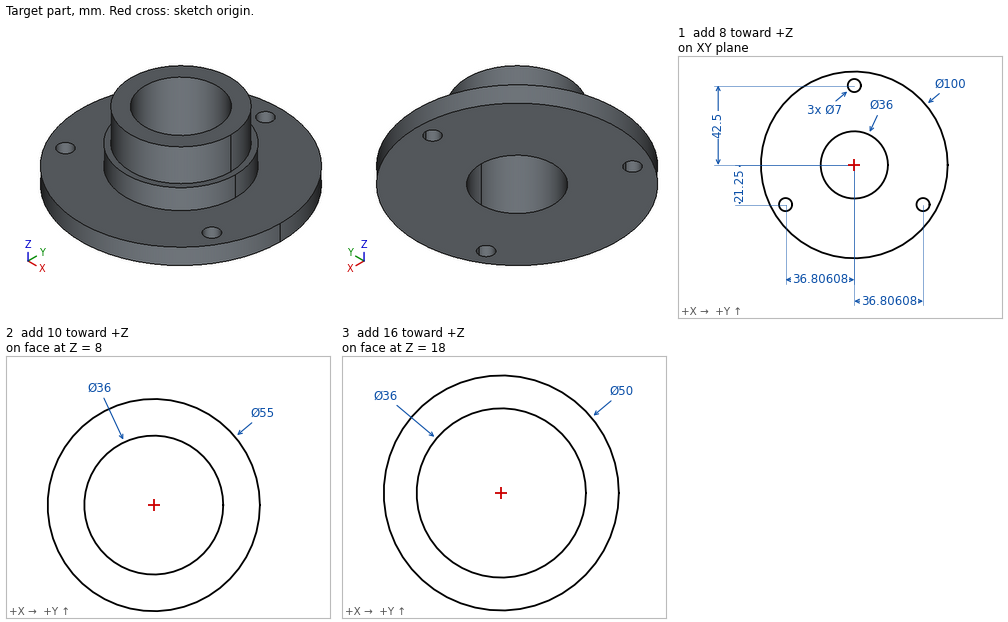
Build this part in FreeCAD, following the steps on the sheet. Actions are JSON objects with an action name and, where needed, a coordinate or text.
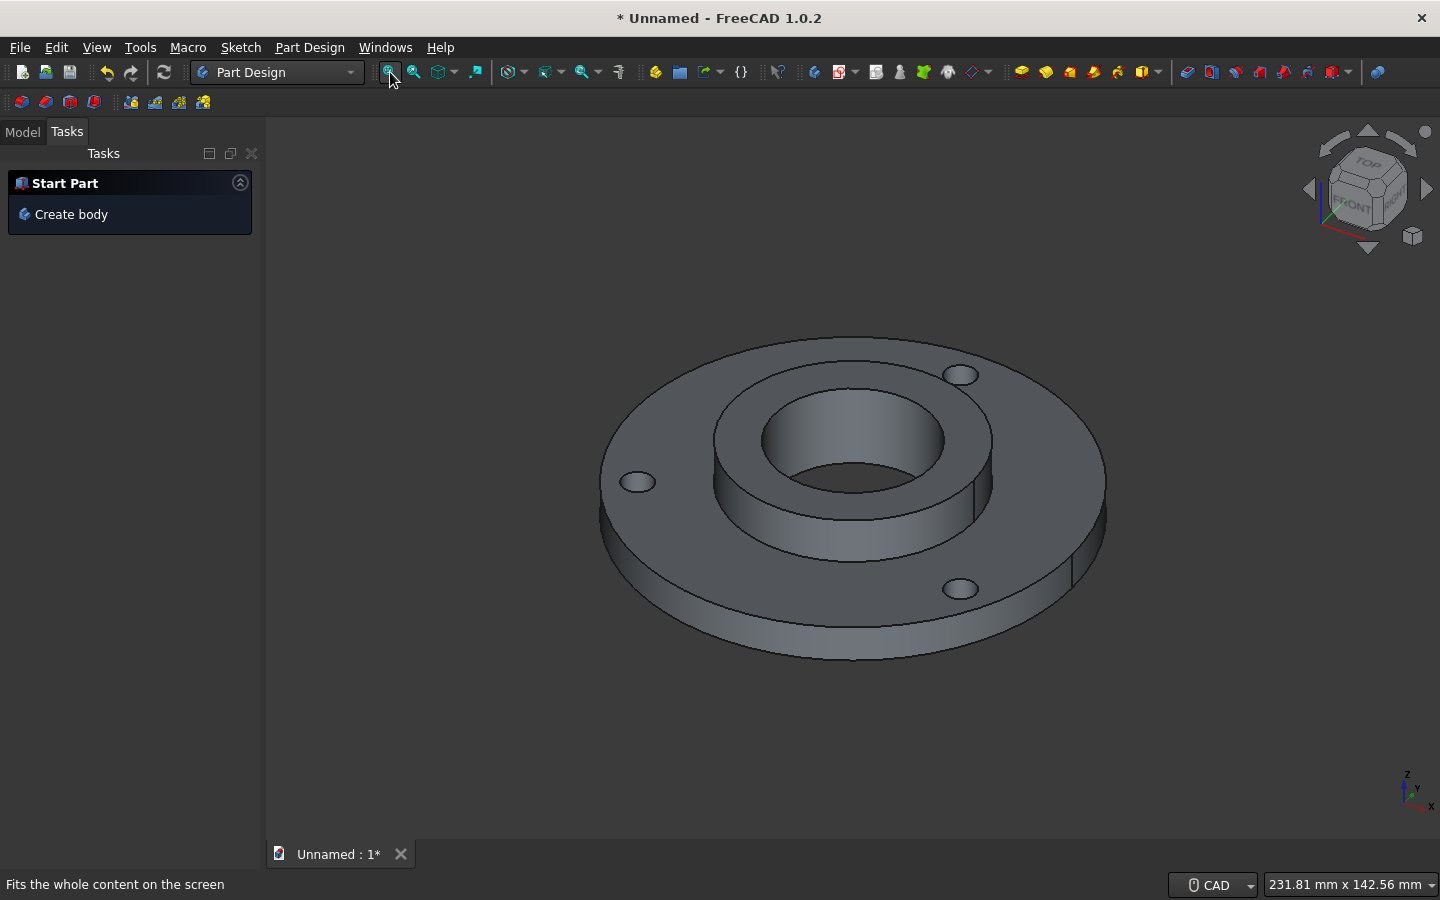
{"action": "left_click", "coordinate": [962, 423]}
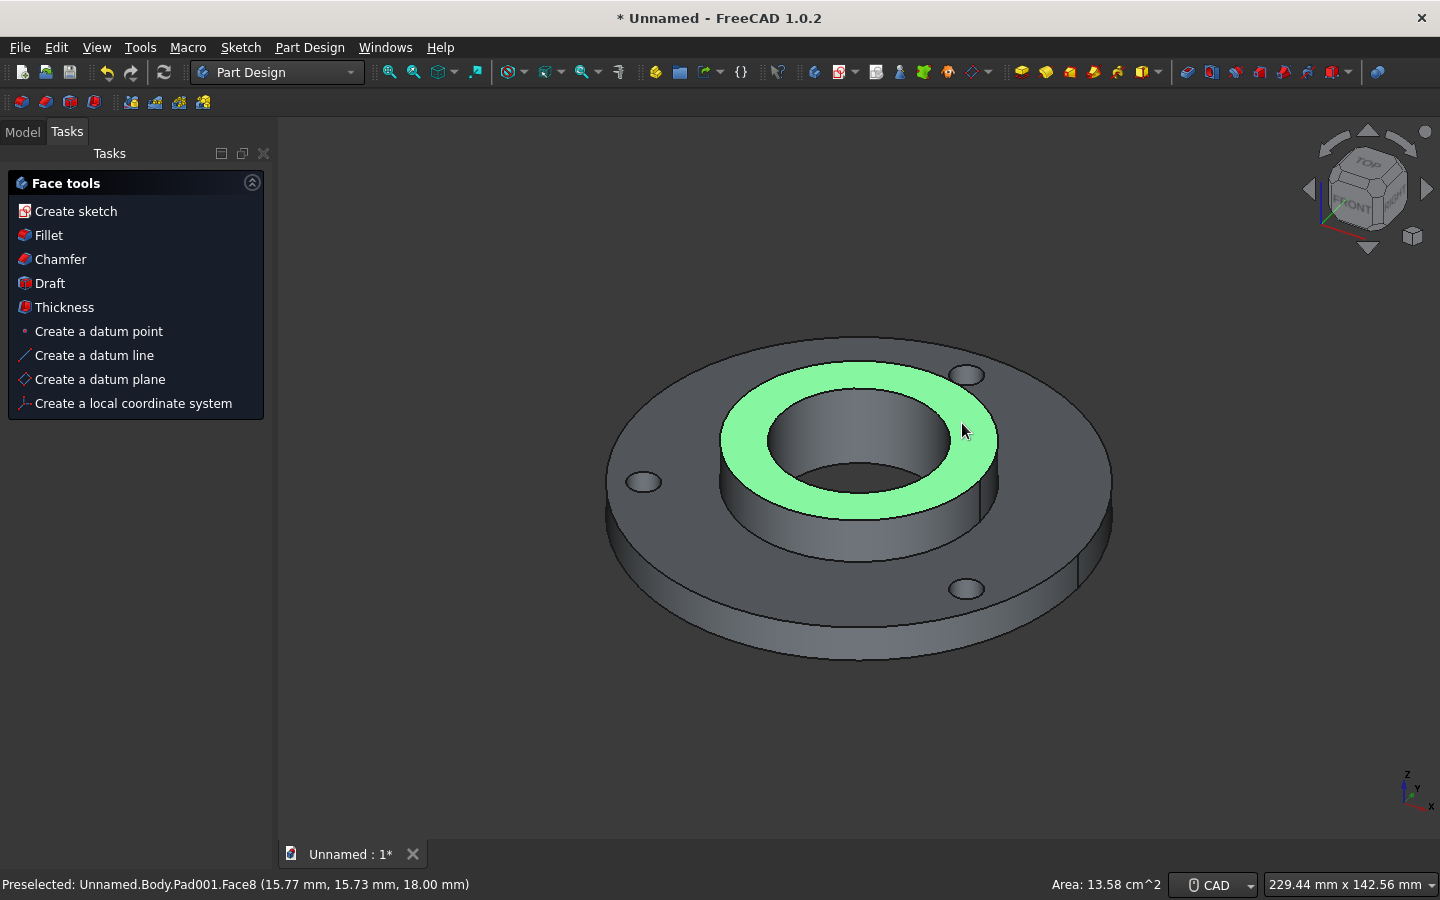
{"action": "left_click", "coordinate": [840, 72]}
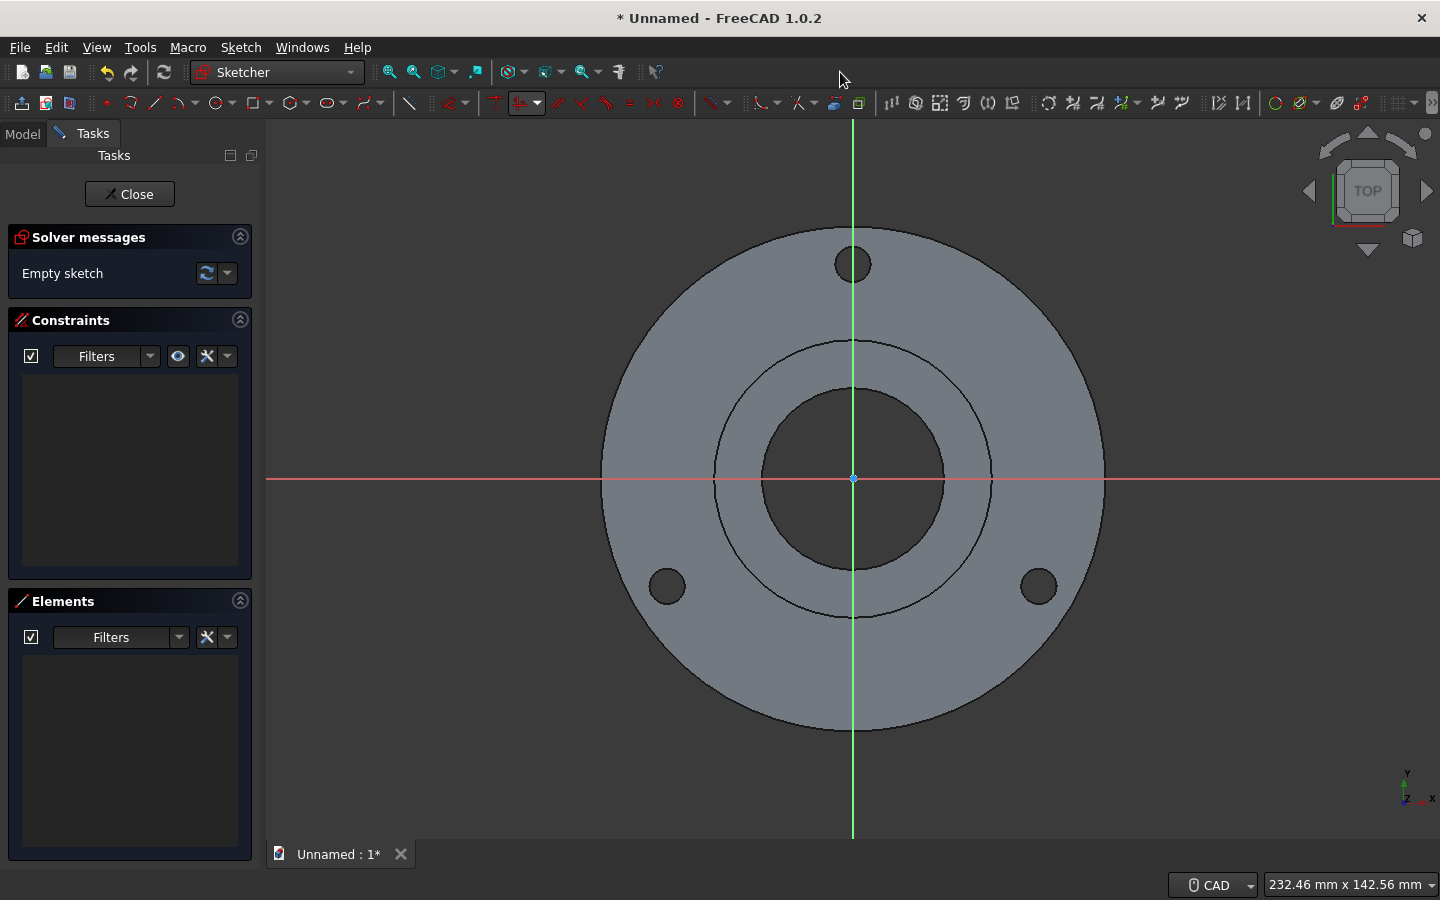
{"action": "scroll", "coordinate": [936, 479], "scroll_direction": "up", "scroll_amount": 3}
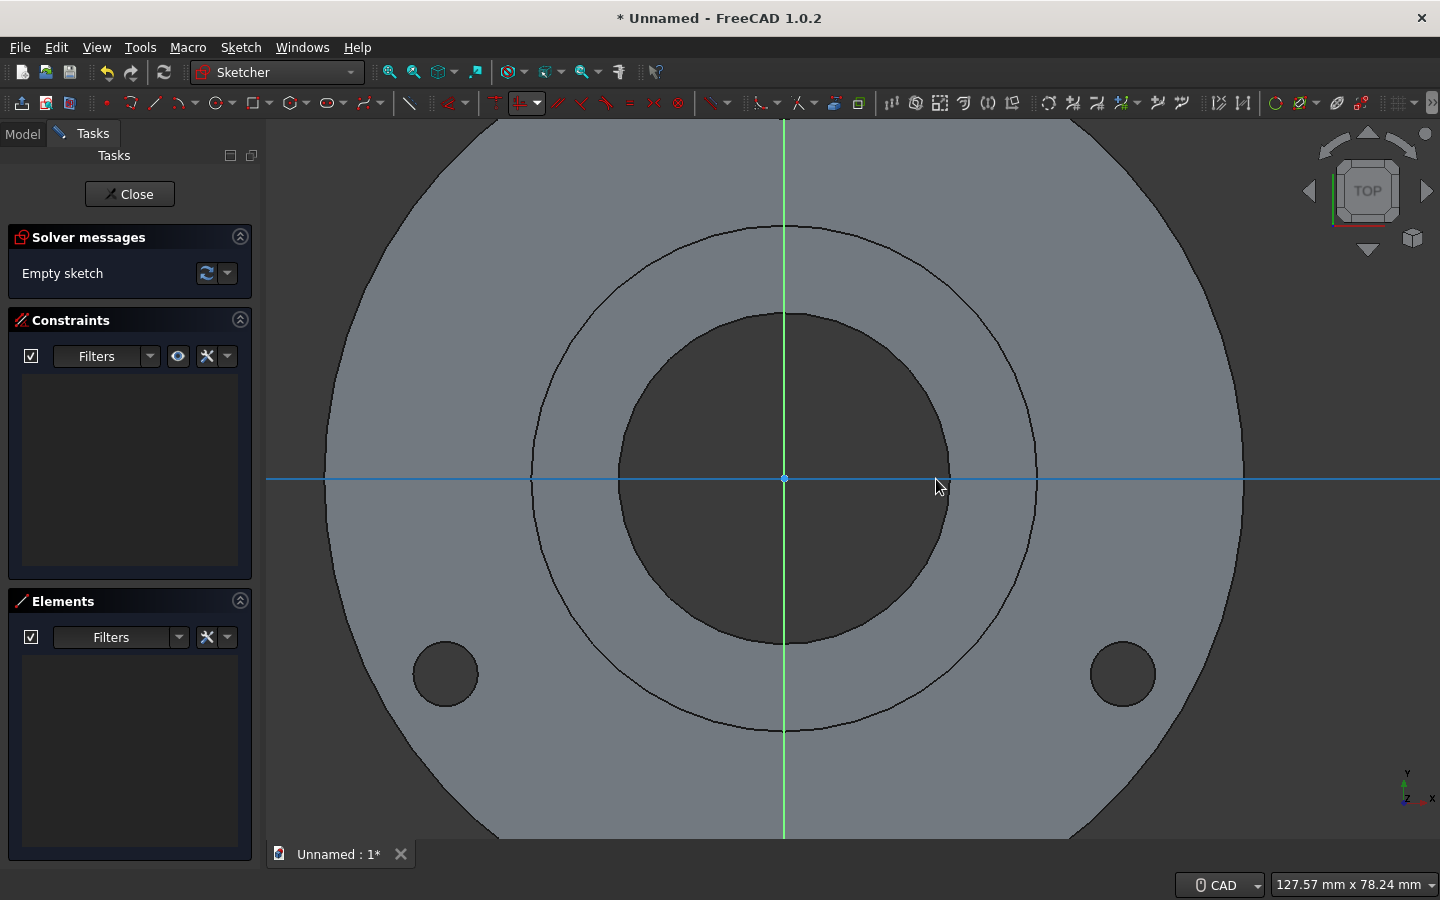
{"action": "left_click", "coordinate": [216, 104]}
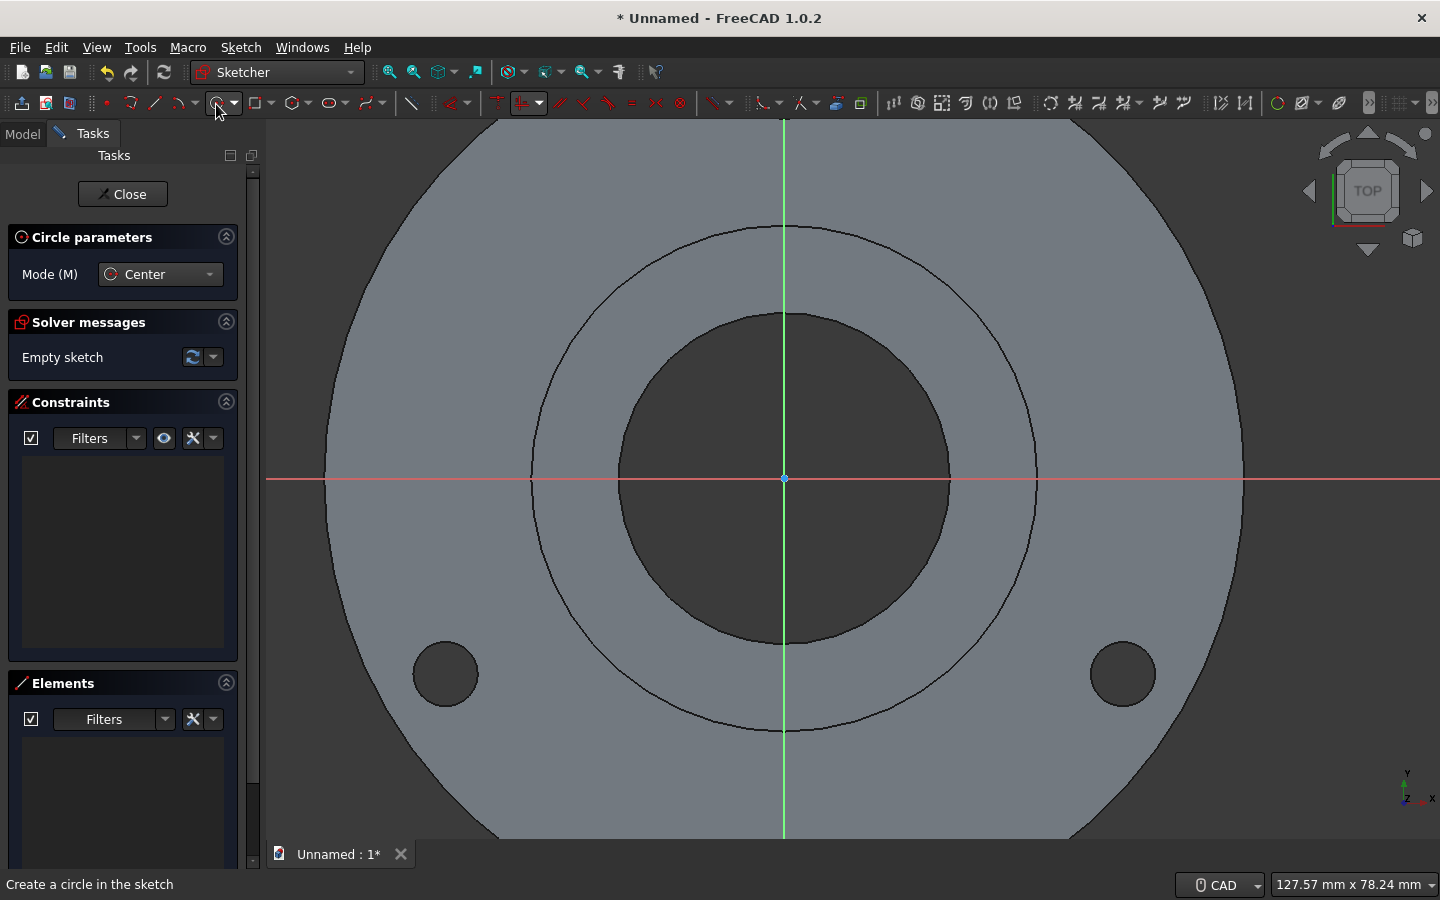
{"action": "left_click", "coordinate": [784, 479]}
{"action": "left_click", "coordinate": [947, 316]}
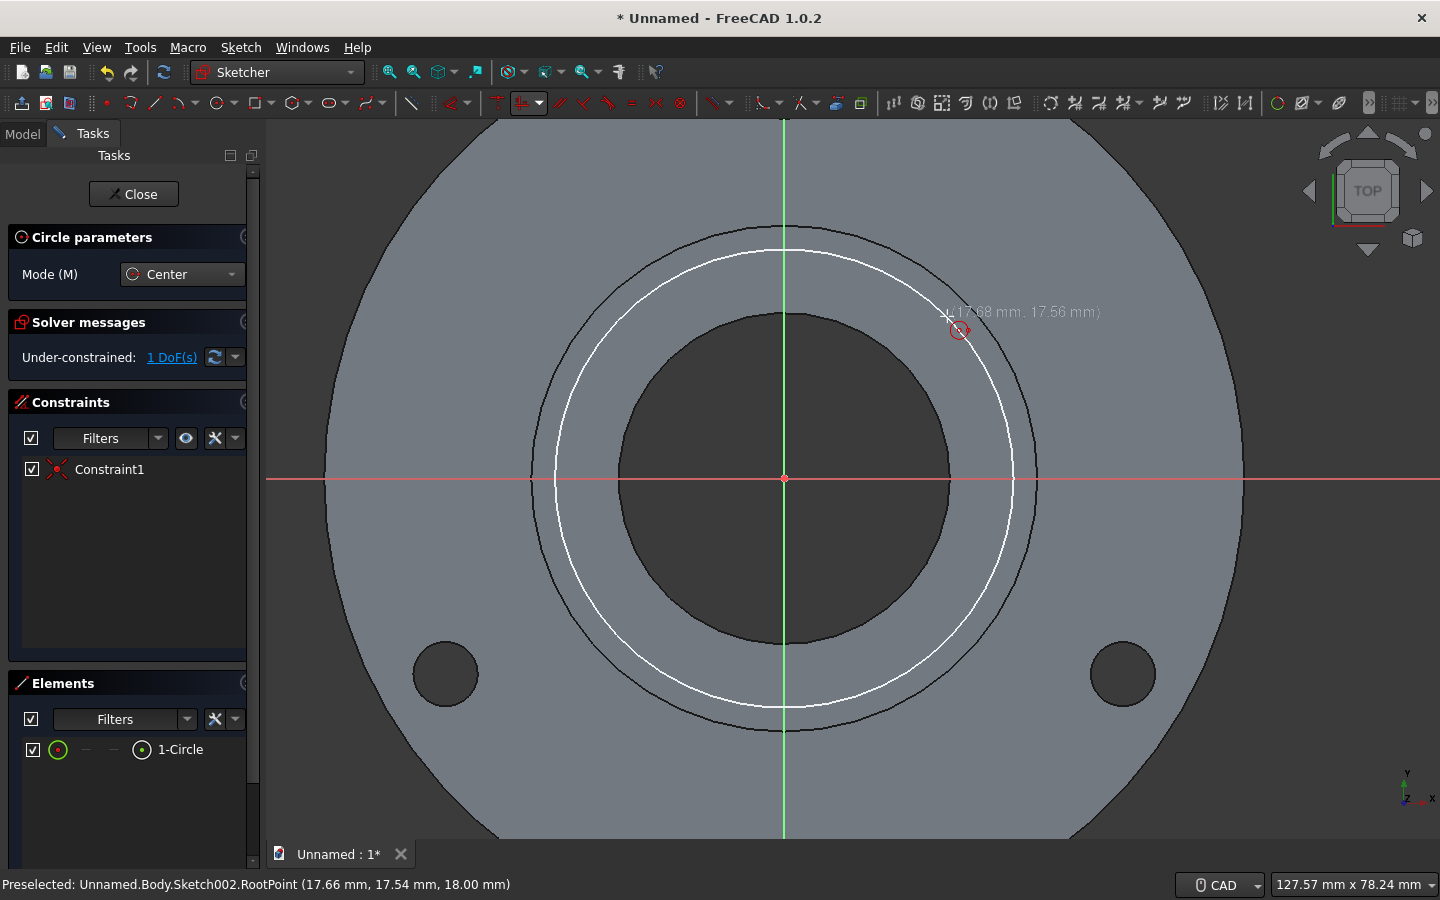
{"action": "left_click", "coordinate": [784, 479]}
{"action": "left_click", "coordinate": [901, 361]}
{"action": "key", "text": "Escape"}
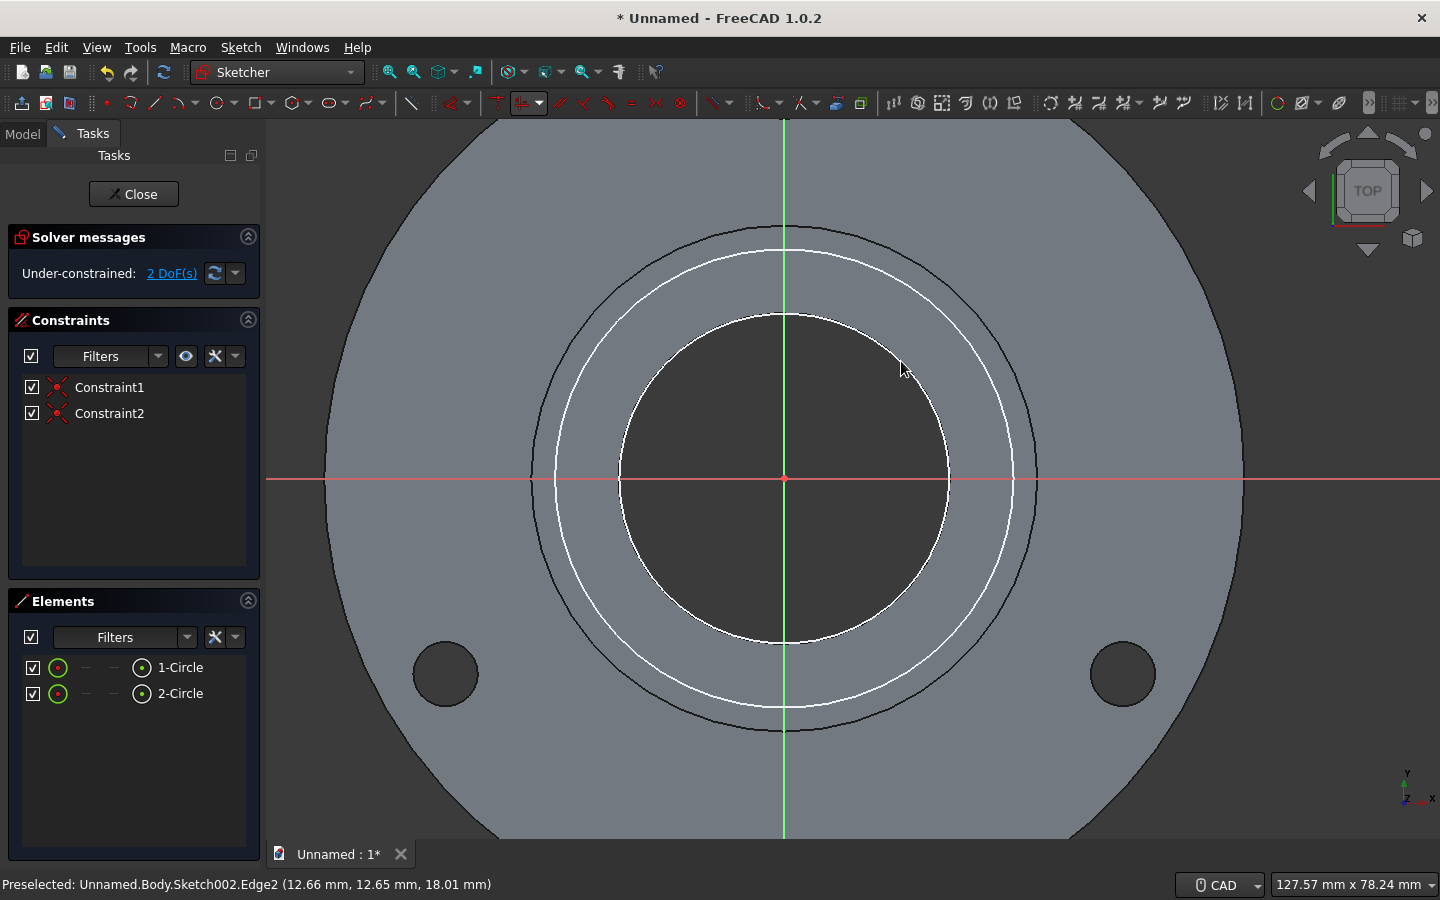
{"action": "left_click", "coordinate": [450, 104]}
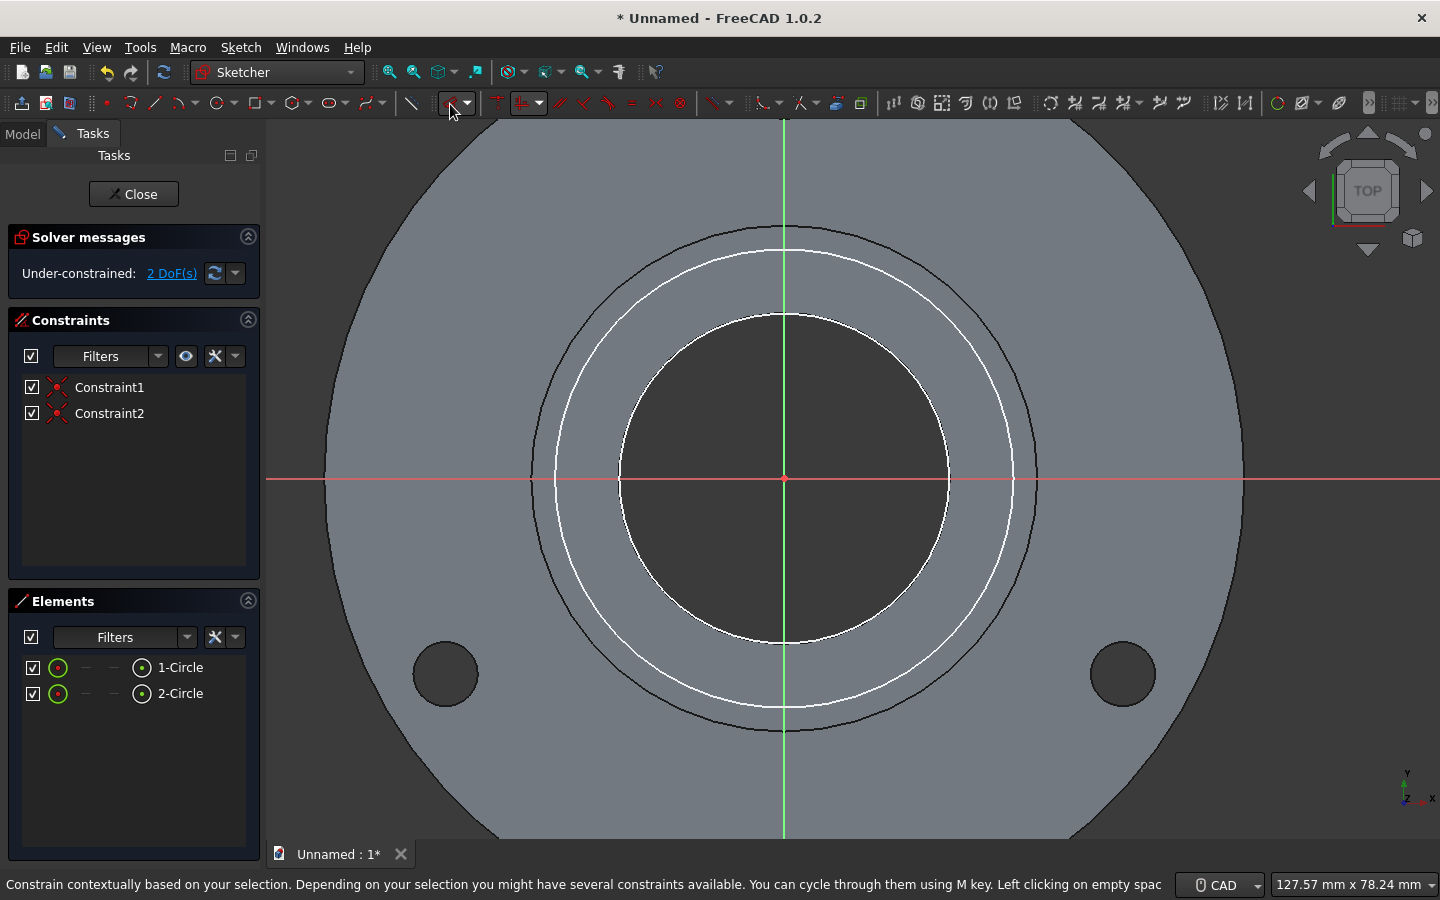
{"action": "left_click", "coordinate": [946, 316]}
{"action": "left_click", "coordinate": [969, 293]}